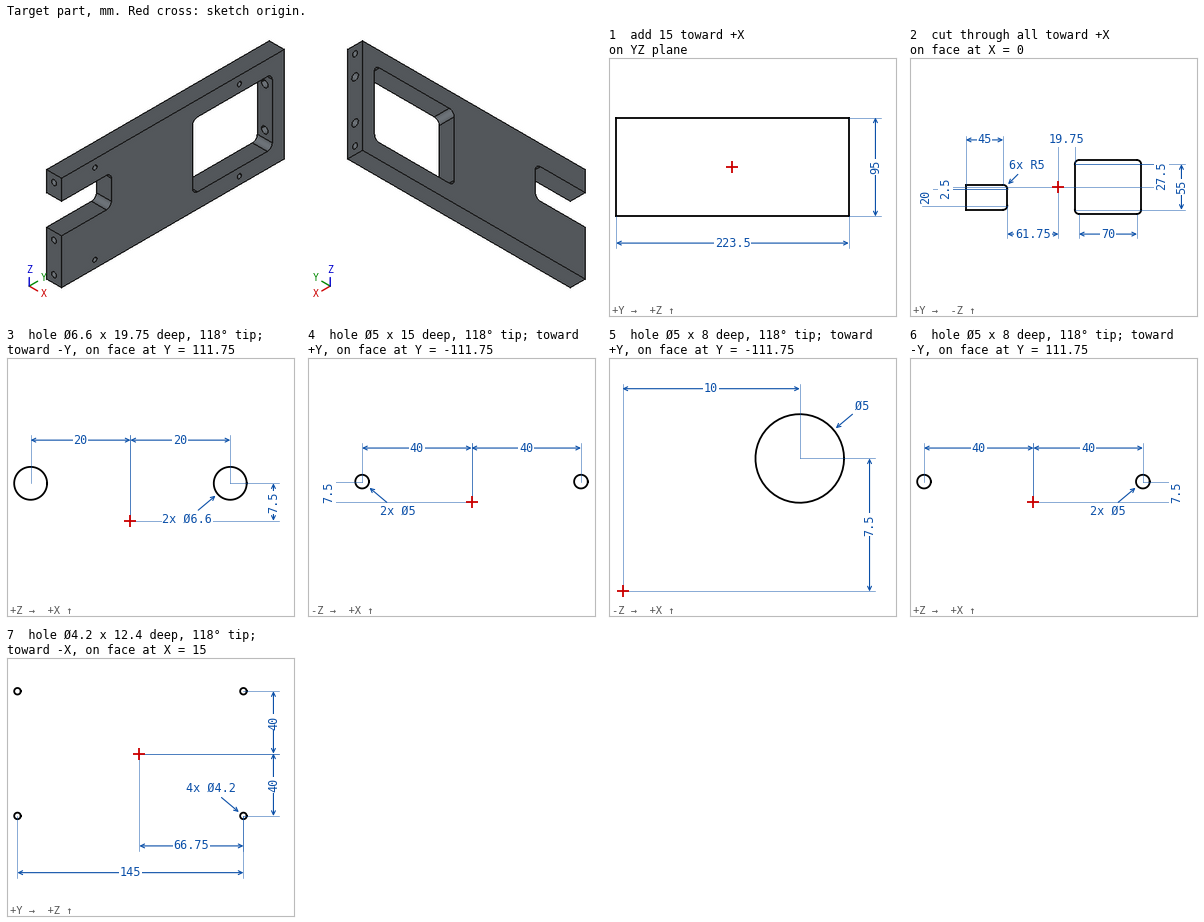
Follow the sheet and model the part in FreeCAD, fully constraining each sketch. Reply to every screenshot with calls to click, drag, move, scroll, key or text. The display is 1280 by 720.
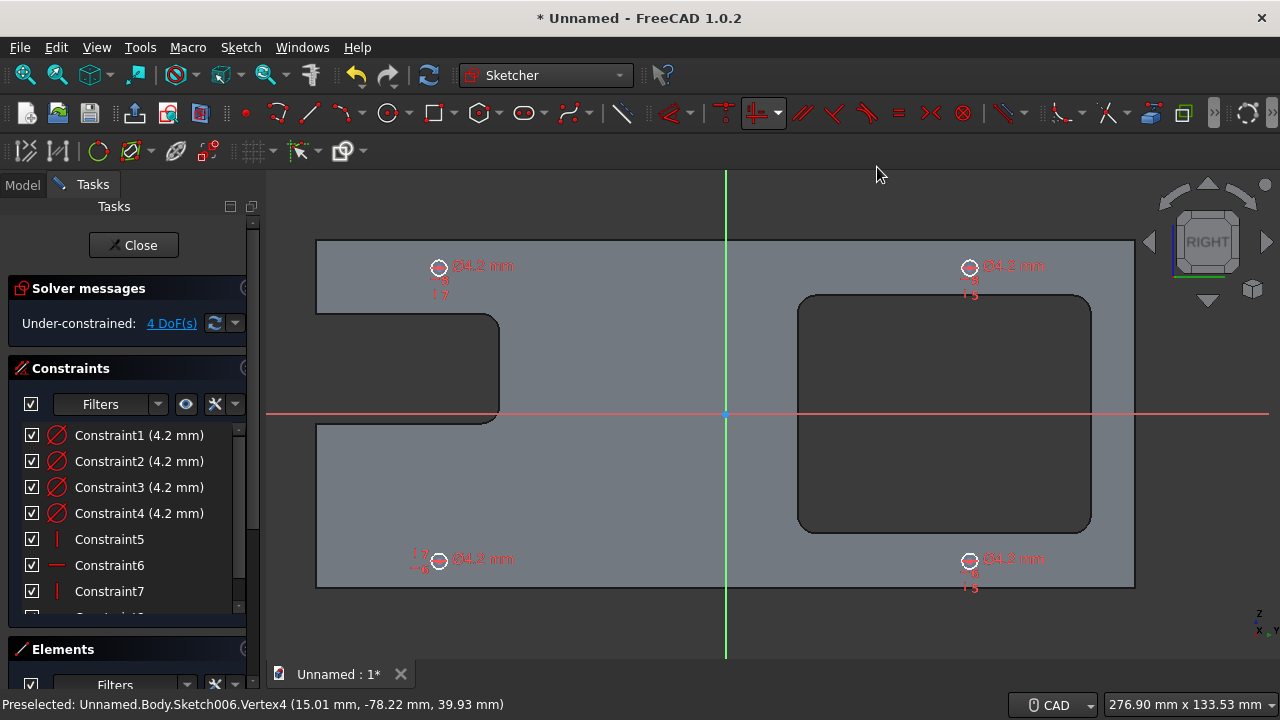
click(670, 114)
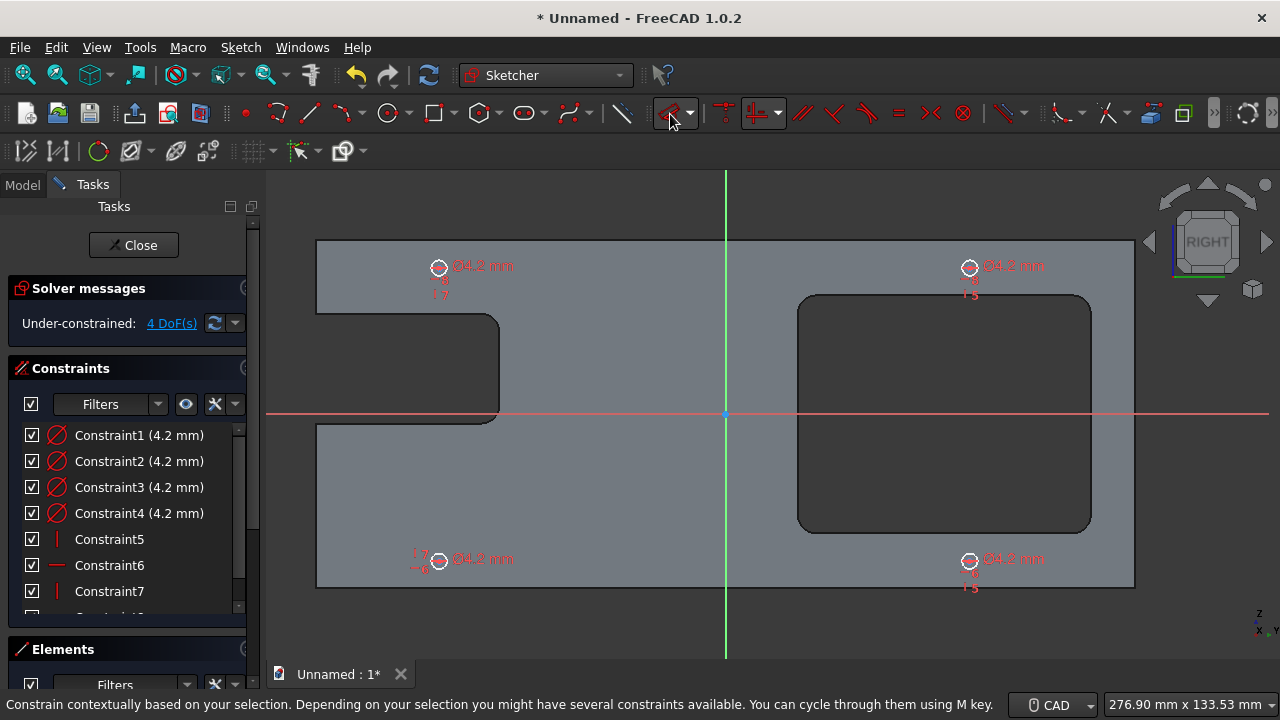
click(970, 561)
click(1004, 488)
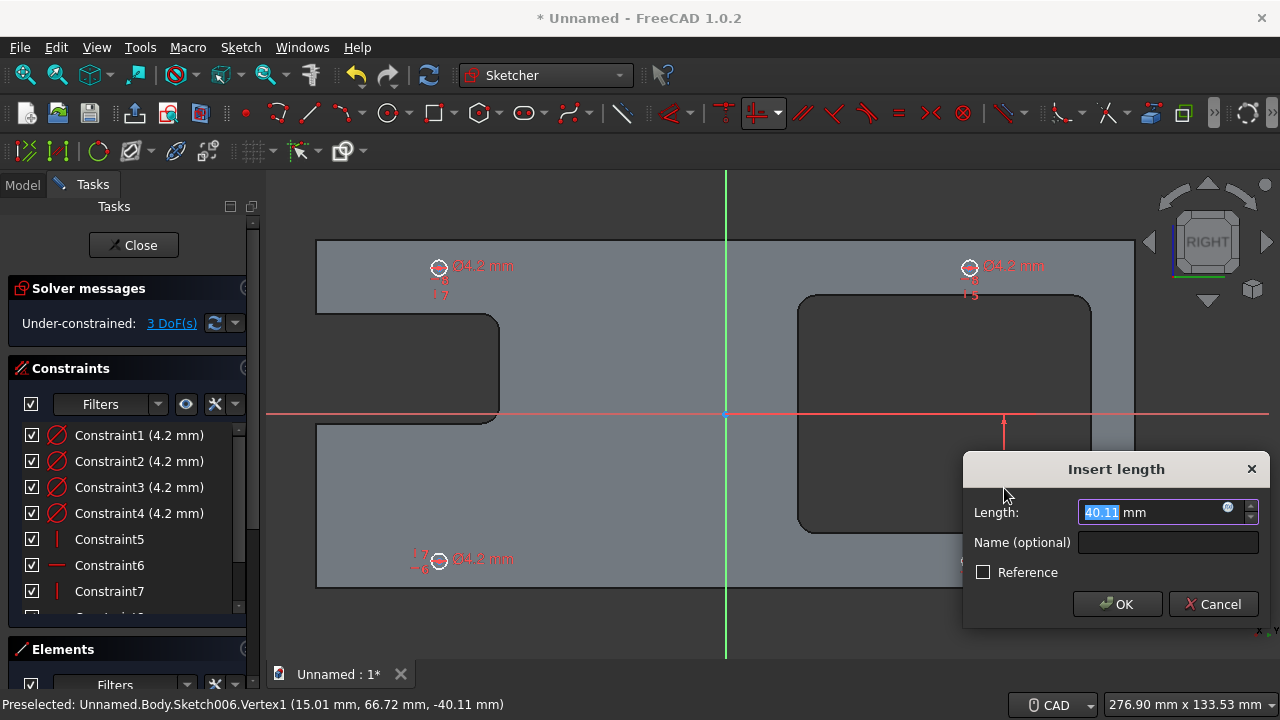
text(40)
key(Return)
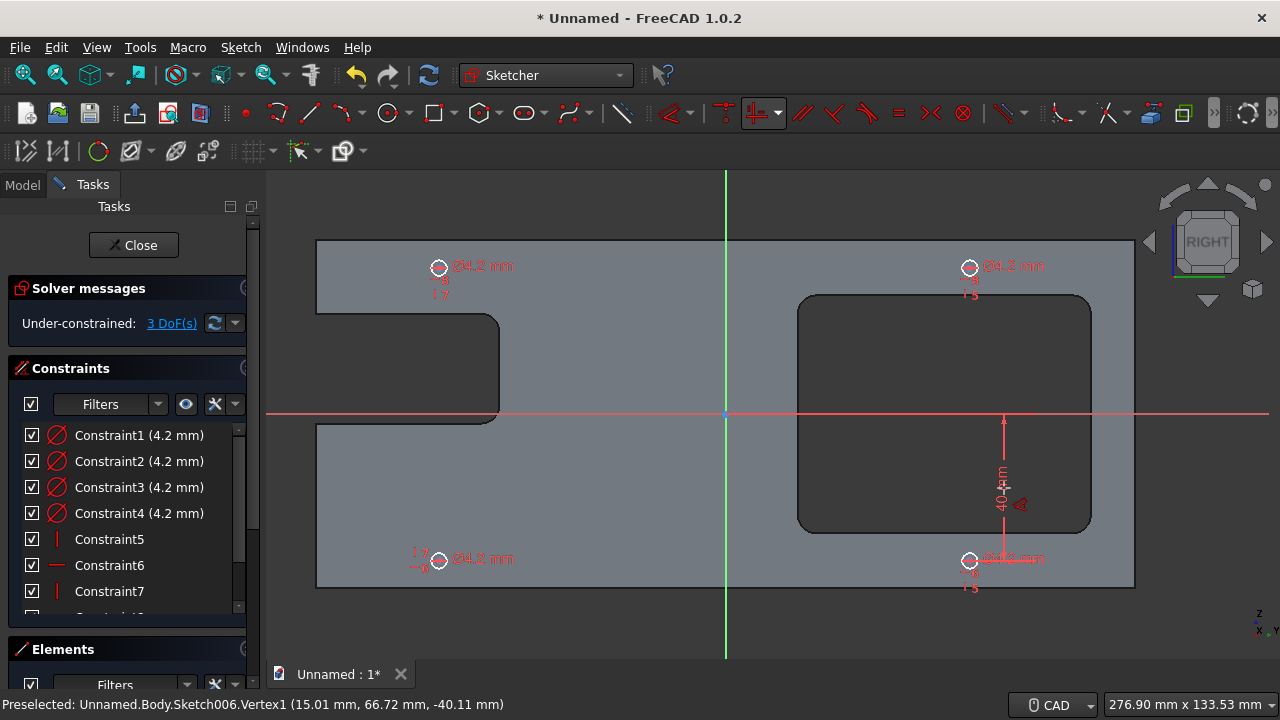
click(970, 268)
click(1004, 341)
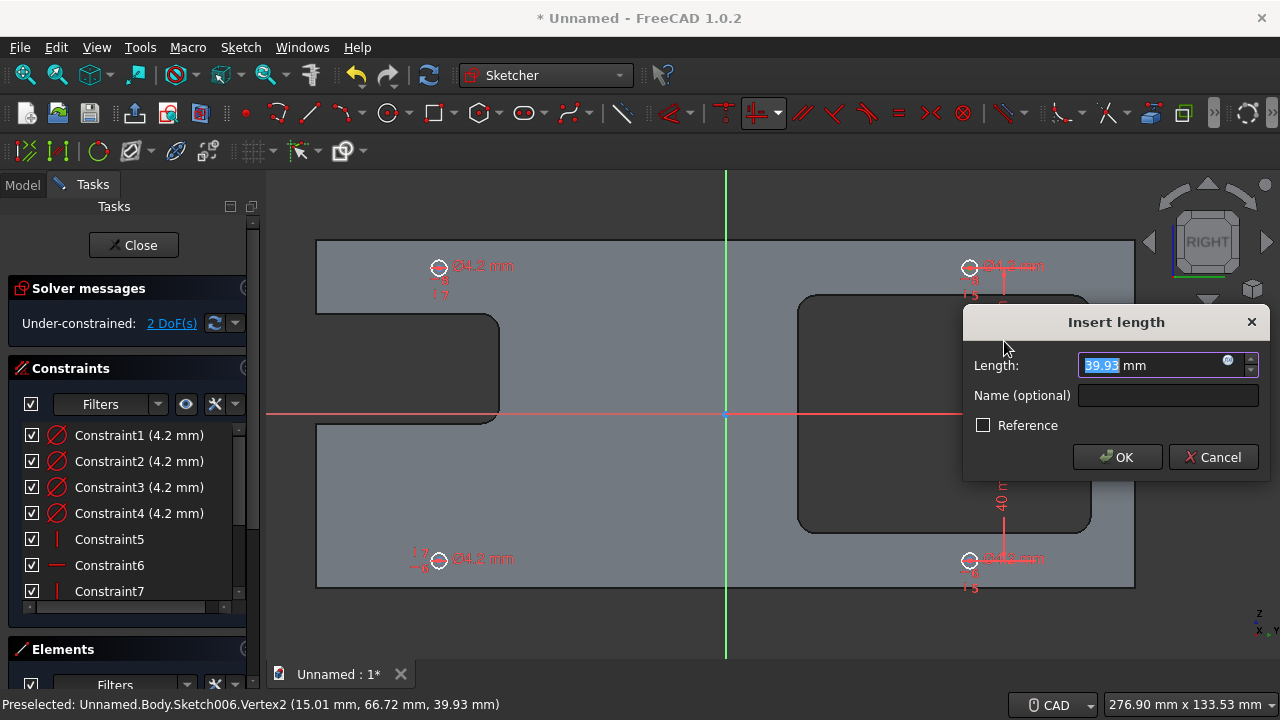
text(40)
key(Return)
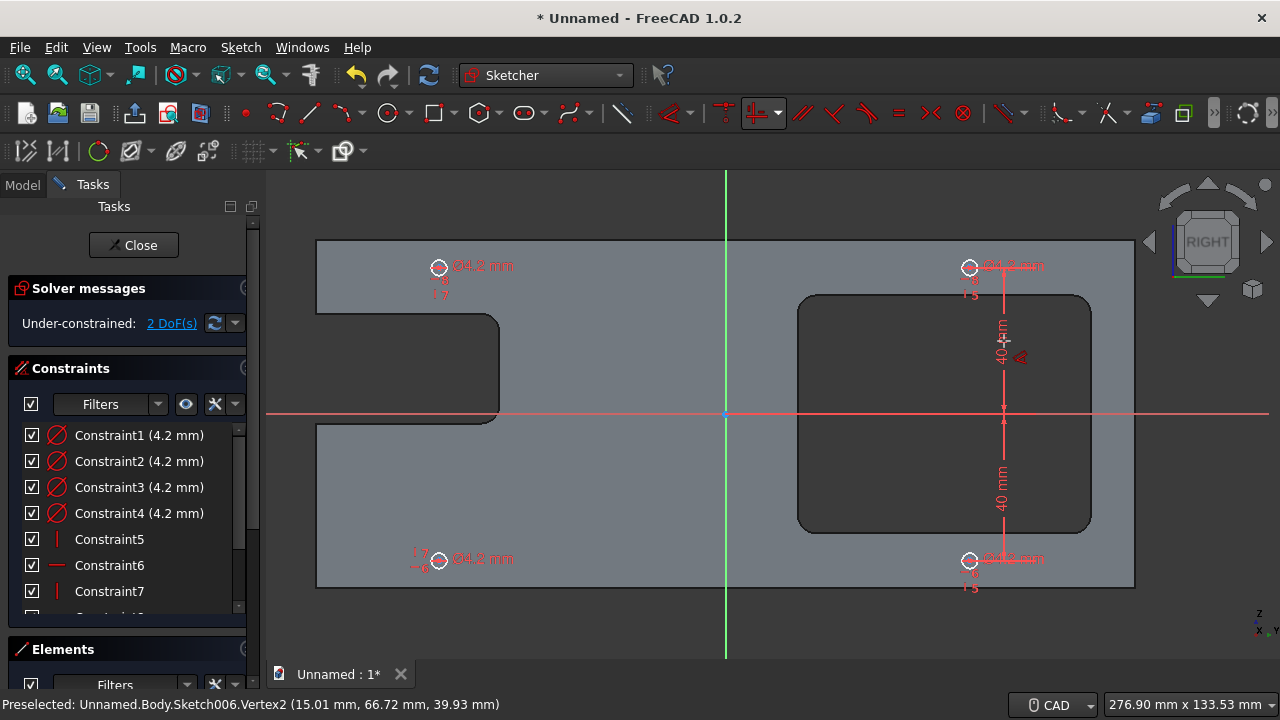
click(970, 561)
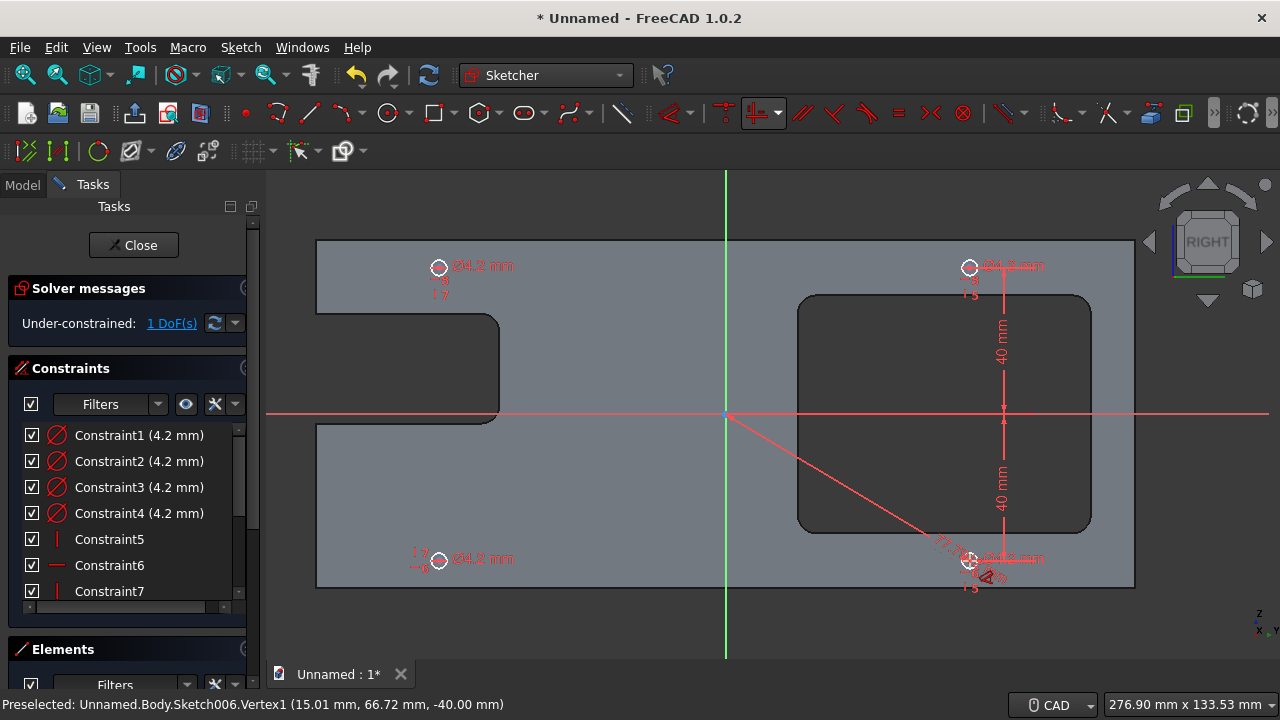
click(439, 561)
click(705, 595)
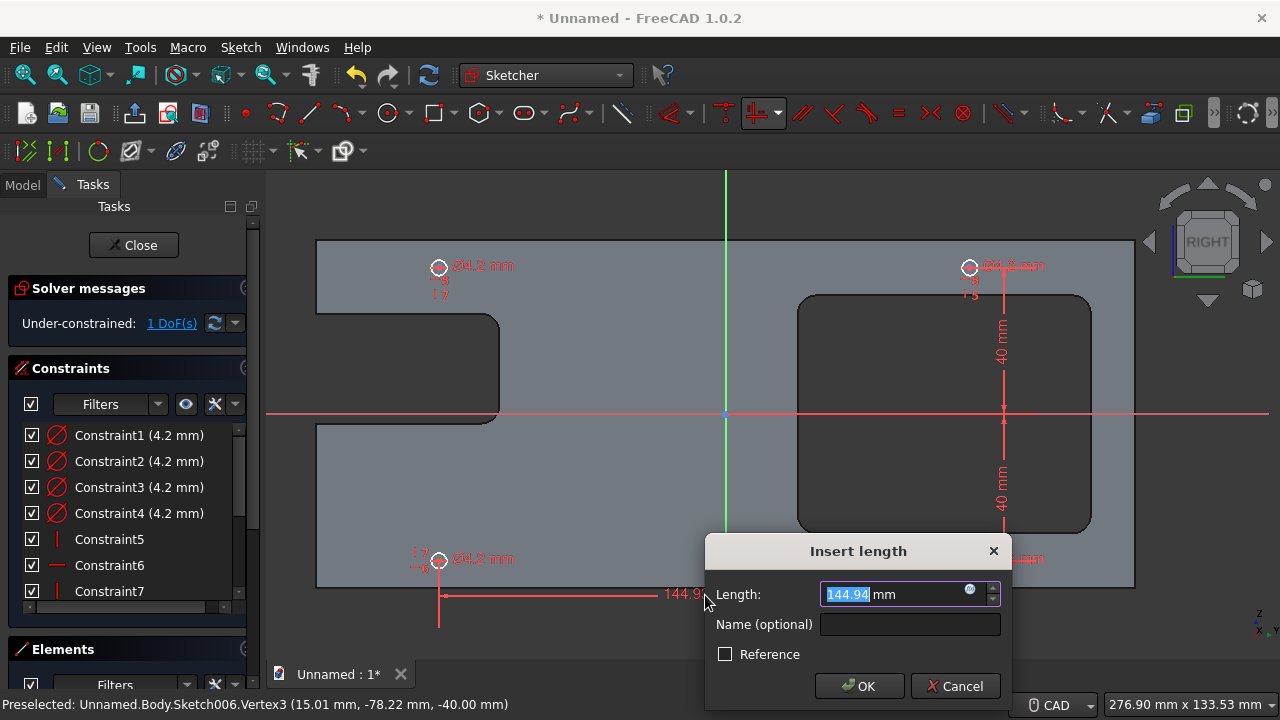
text(145)
key(Return)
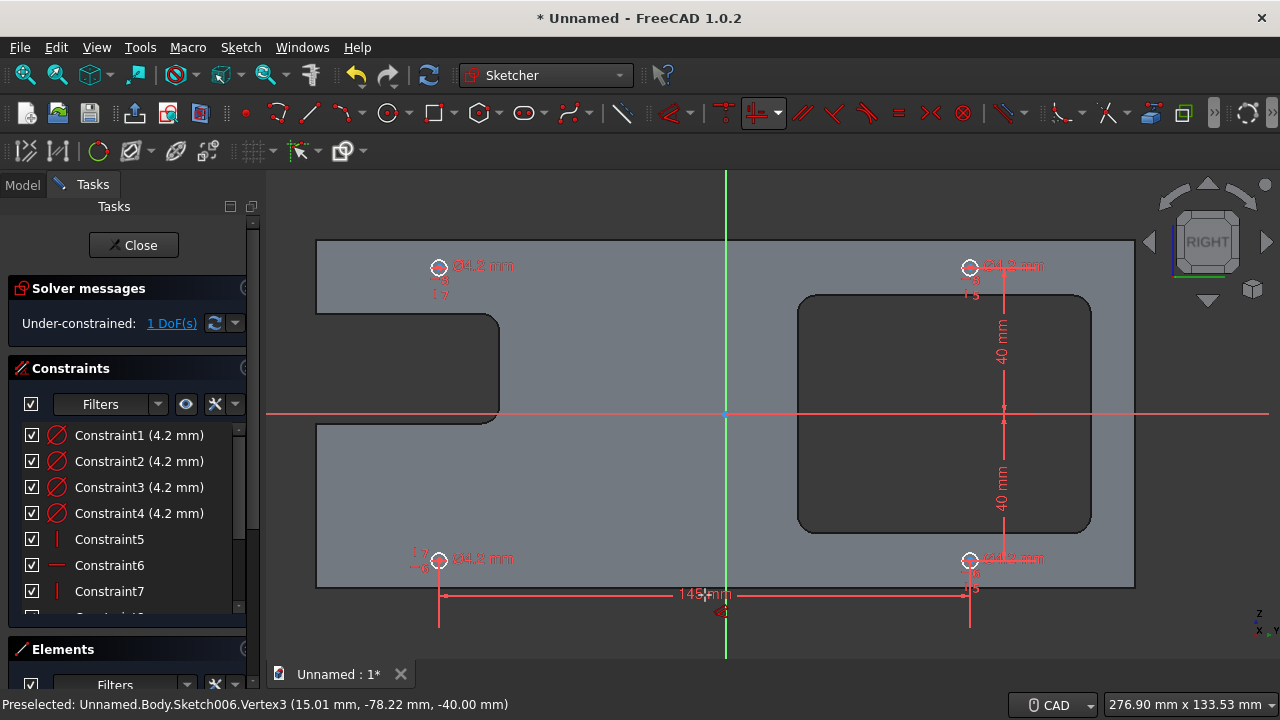
click(970, 561)
click(848, 595)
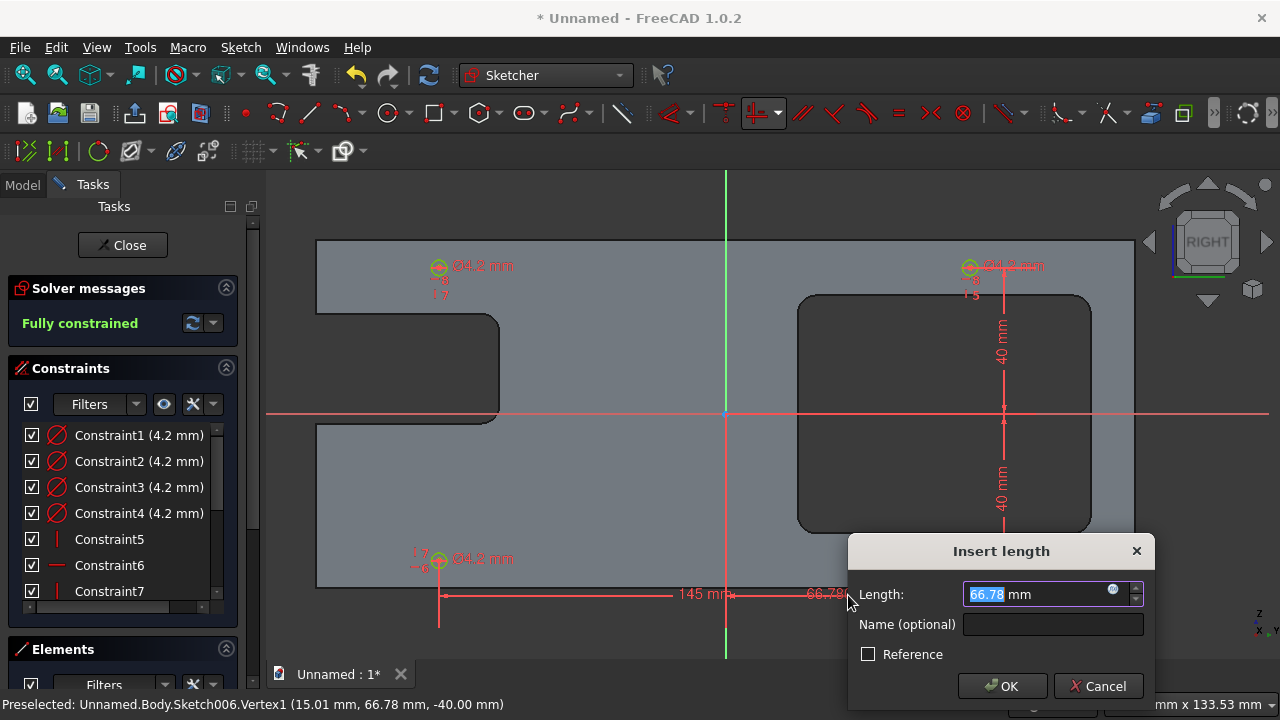
text(66.75)
key(Return)
key(Escape)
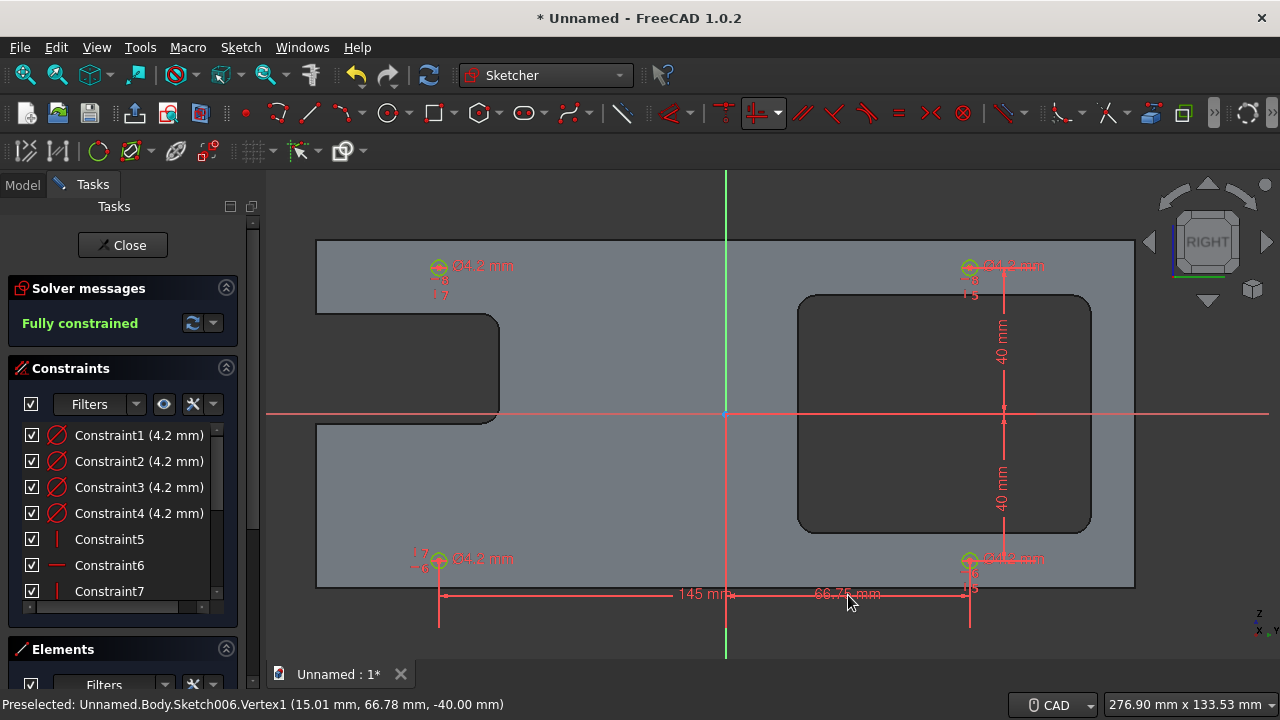
click(123, 245)